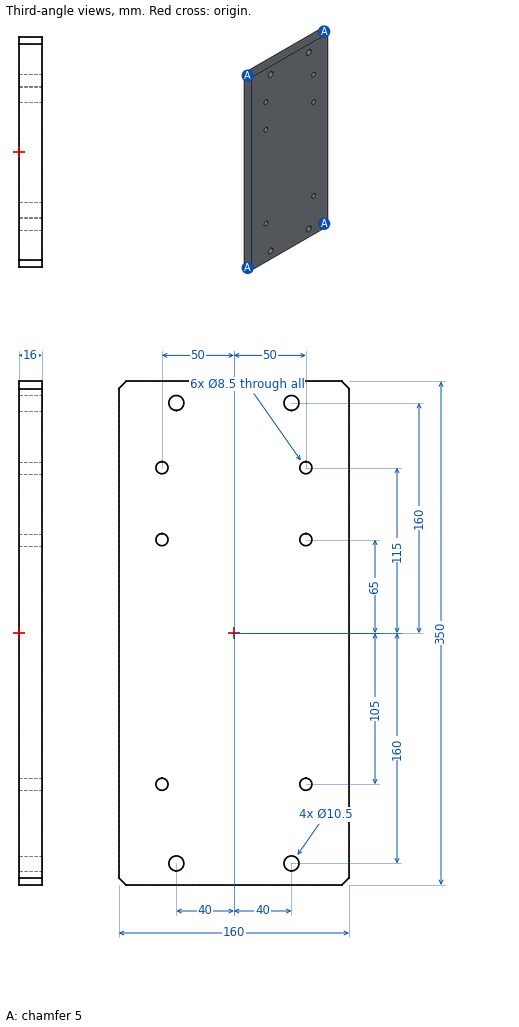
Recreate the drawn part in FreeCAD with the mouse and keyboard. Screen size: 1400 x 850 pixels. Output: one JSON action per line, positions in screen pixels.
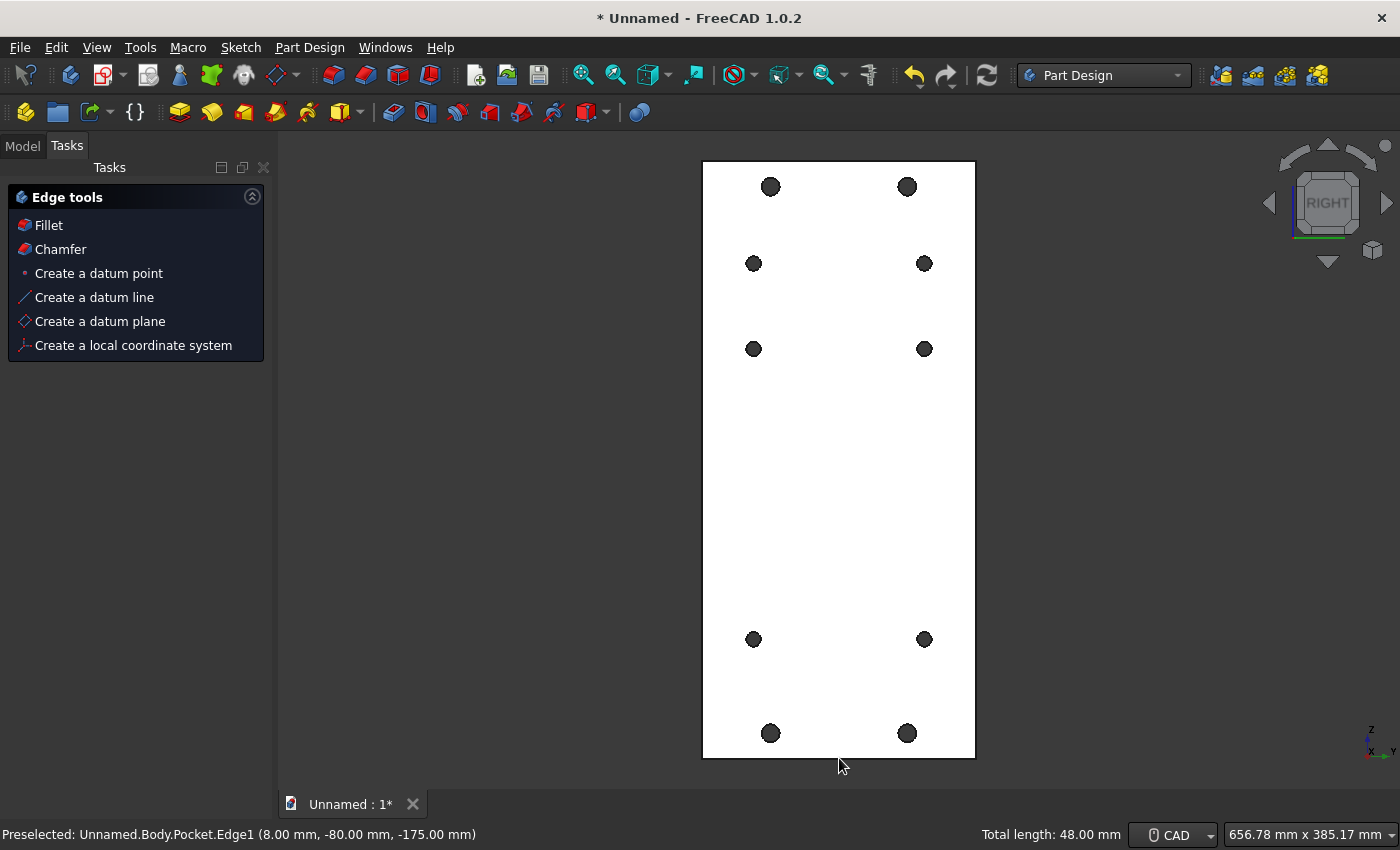
{"action": "key", "text": "5"}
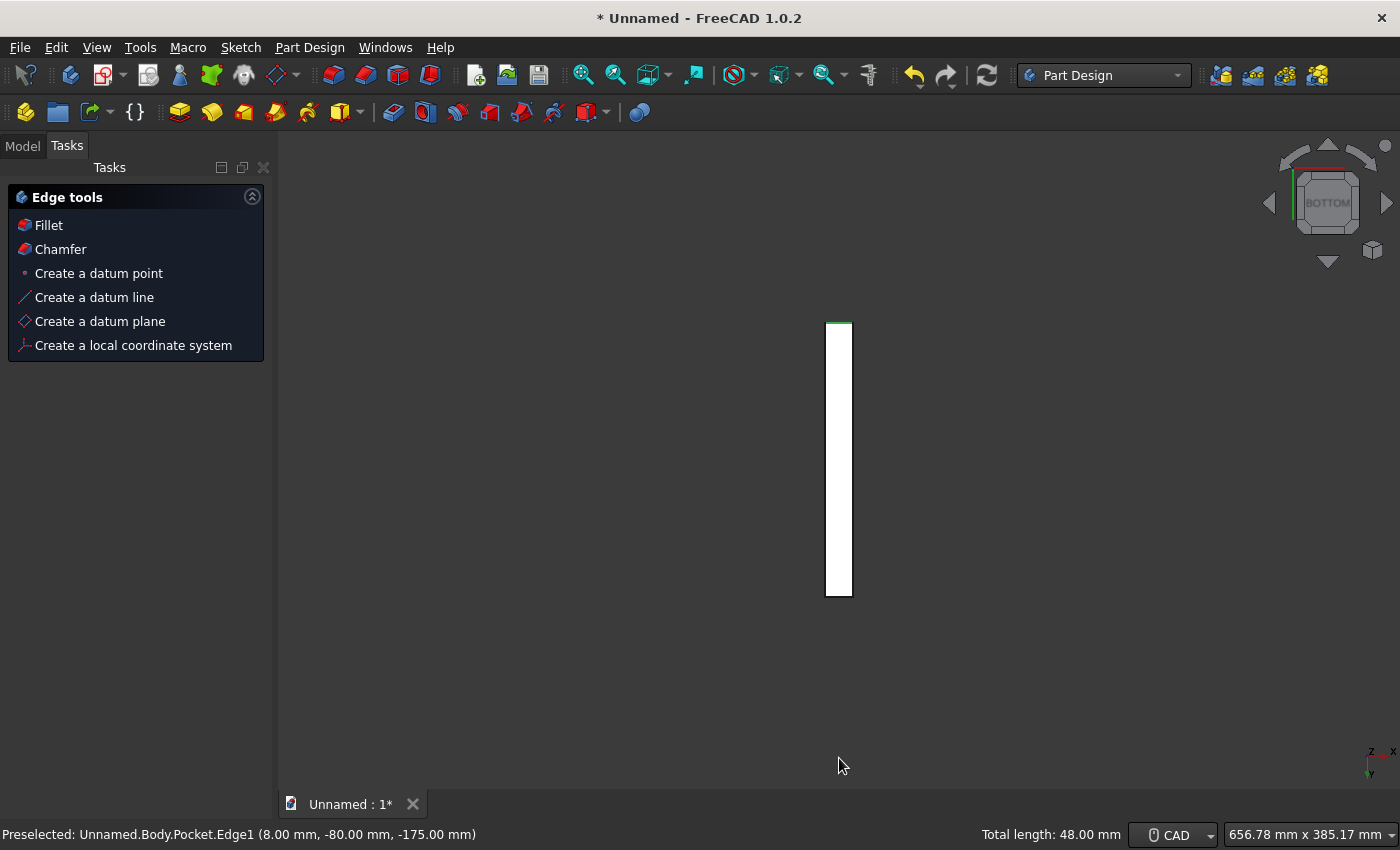
{"action": "key", "text": "v f"}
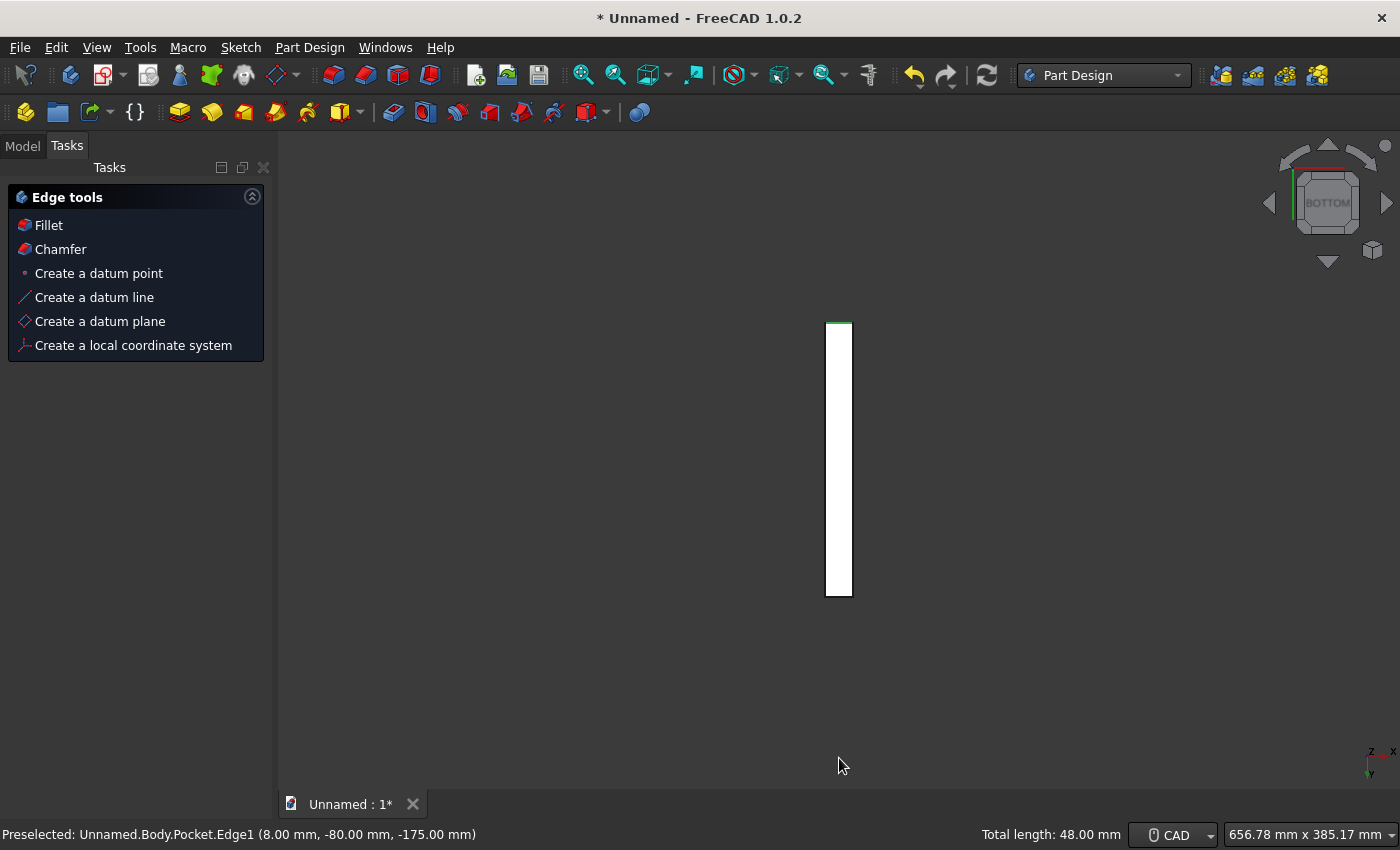
{"action": "left_click", "coordinate": [839, 596], "text": "ctrl"}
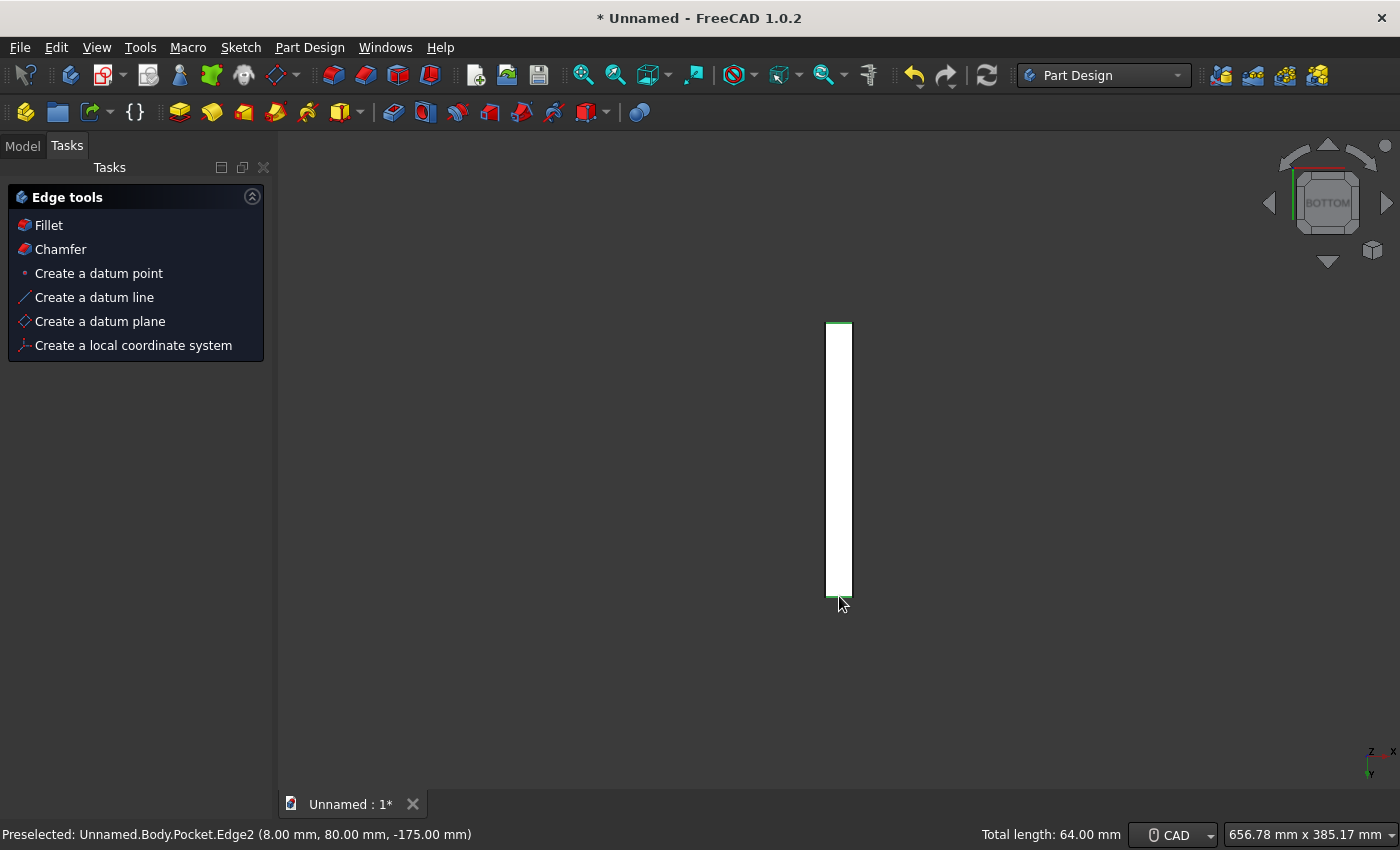
{"action": "left_click", "coordinate": [366, 76]}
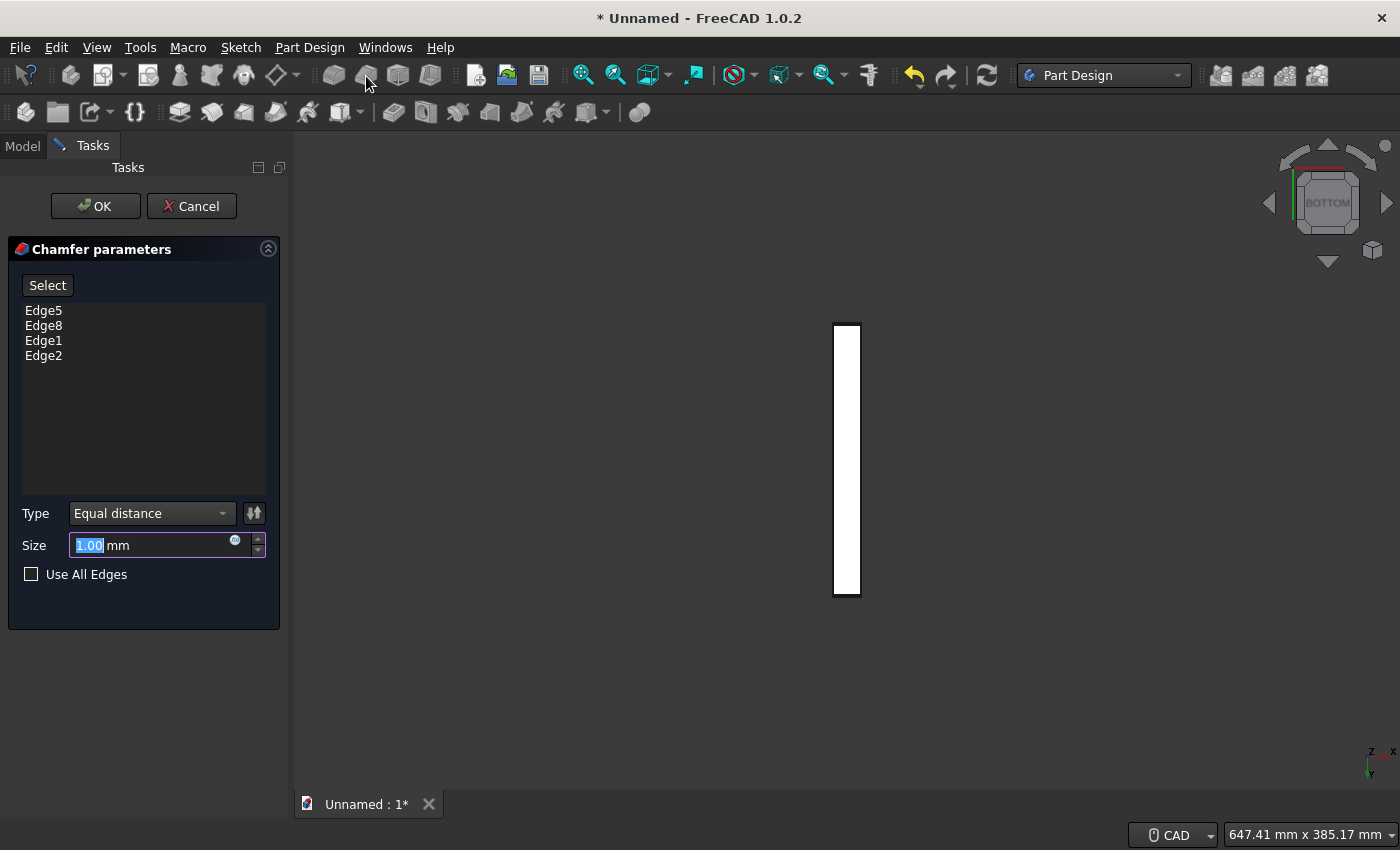
{"action": "type", "text": "5"}
{"action": "key", "text": "Tab"}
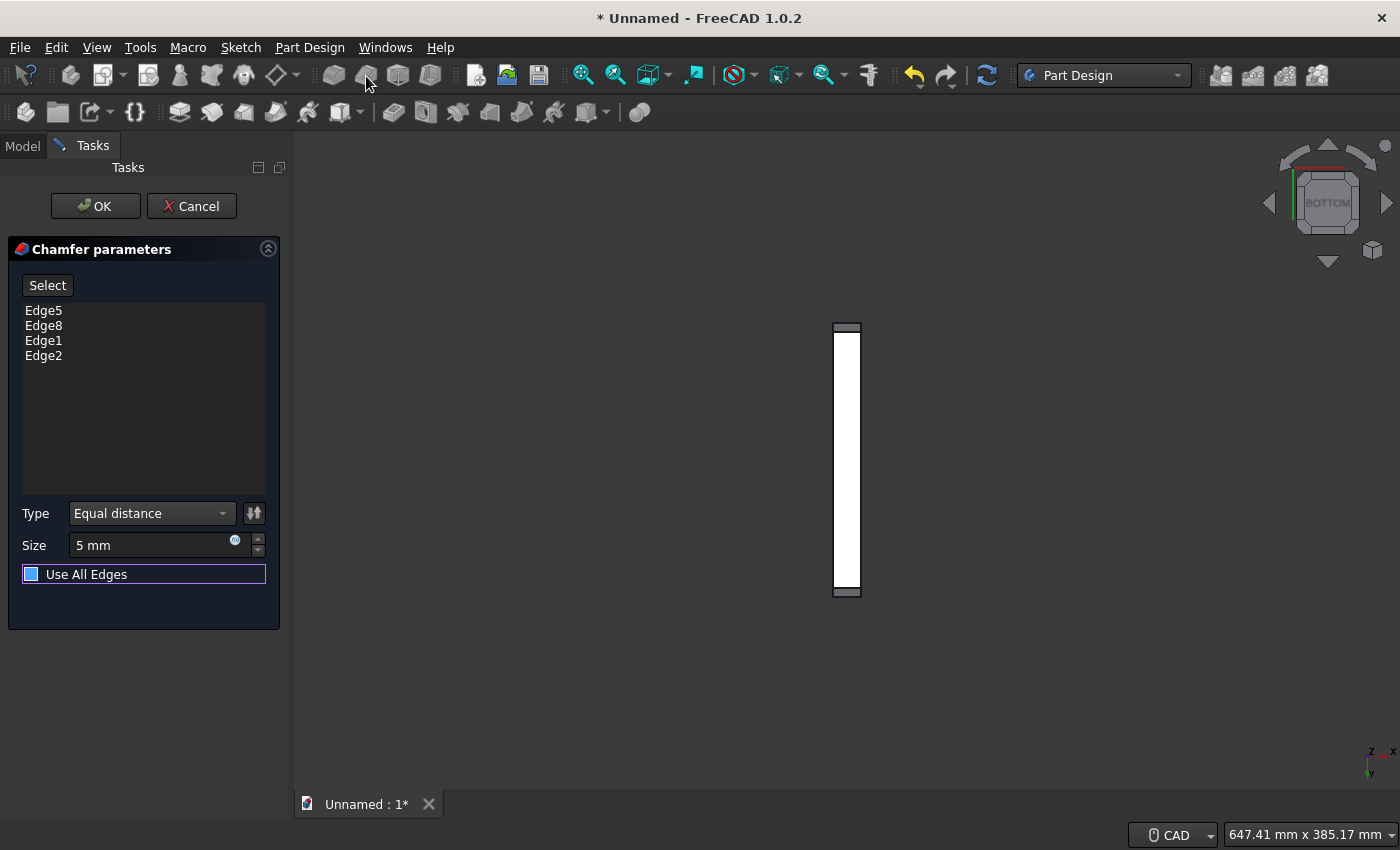
{"action": "left_click", "coordinate": [96, 206]}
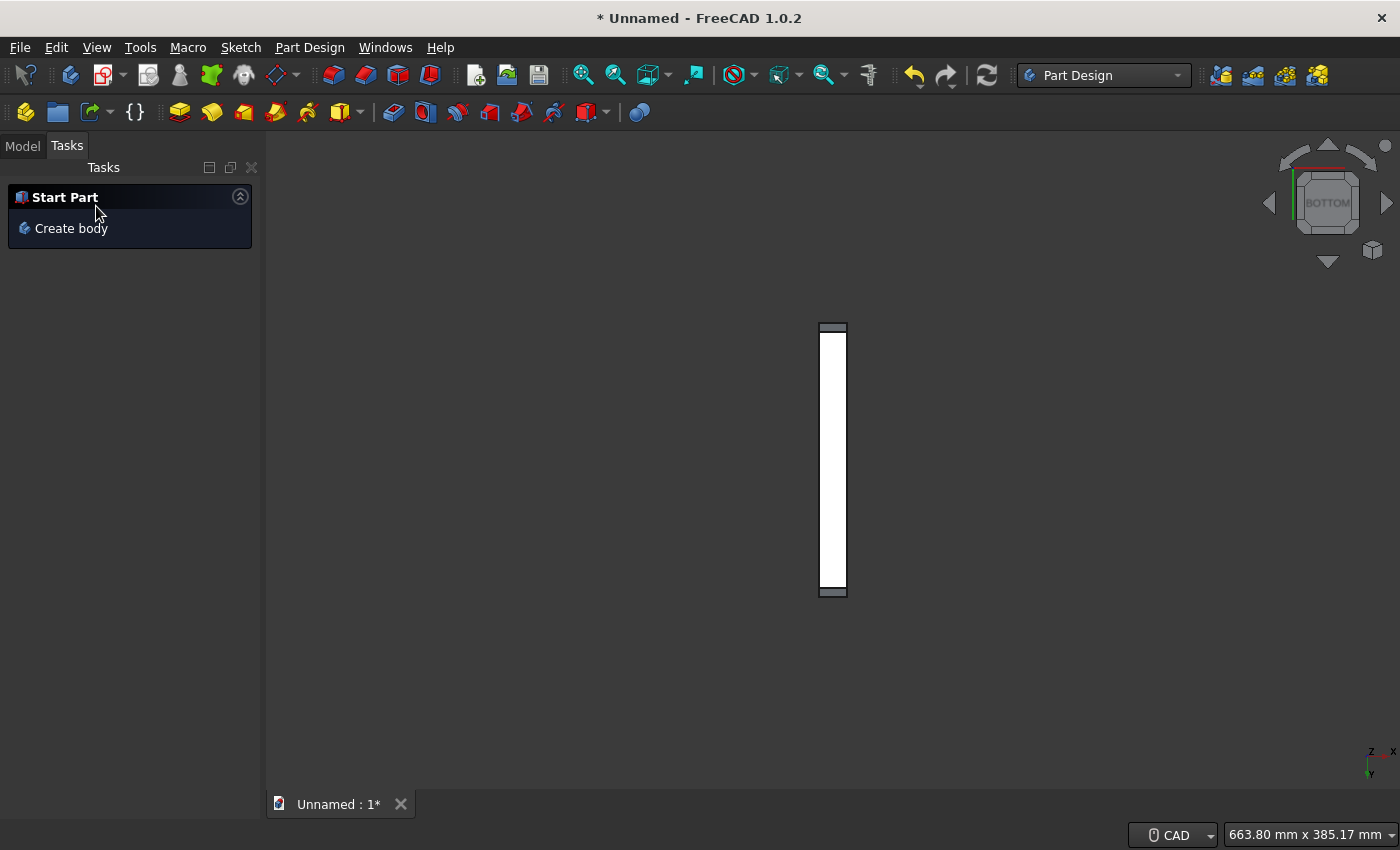
{"action": "key", "text": "0"}